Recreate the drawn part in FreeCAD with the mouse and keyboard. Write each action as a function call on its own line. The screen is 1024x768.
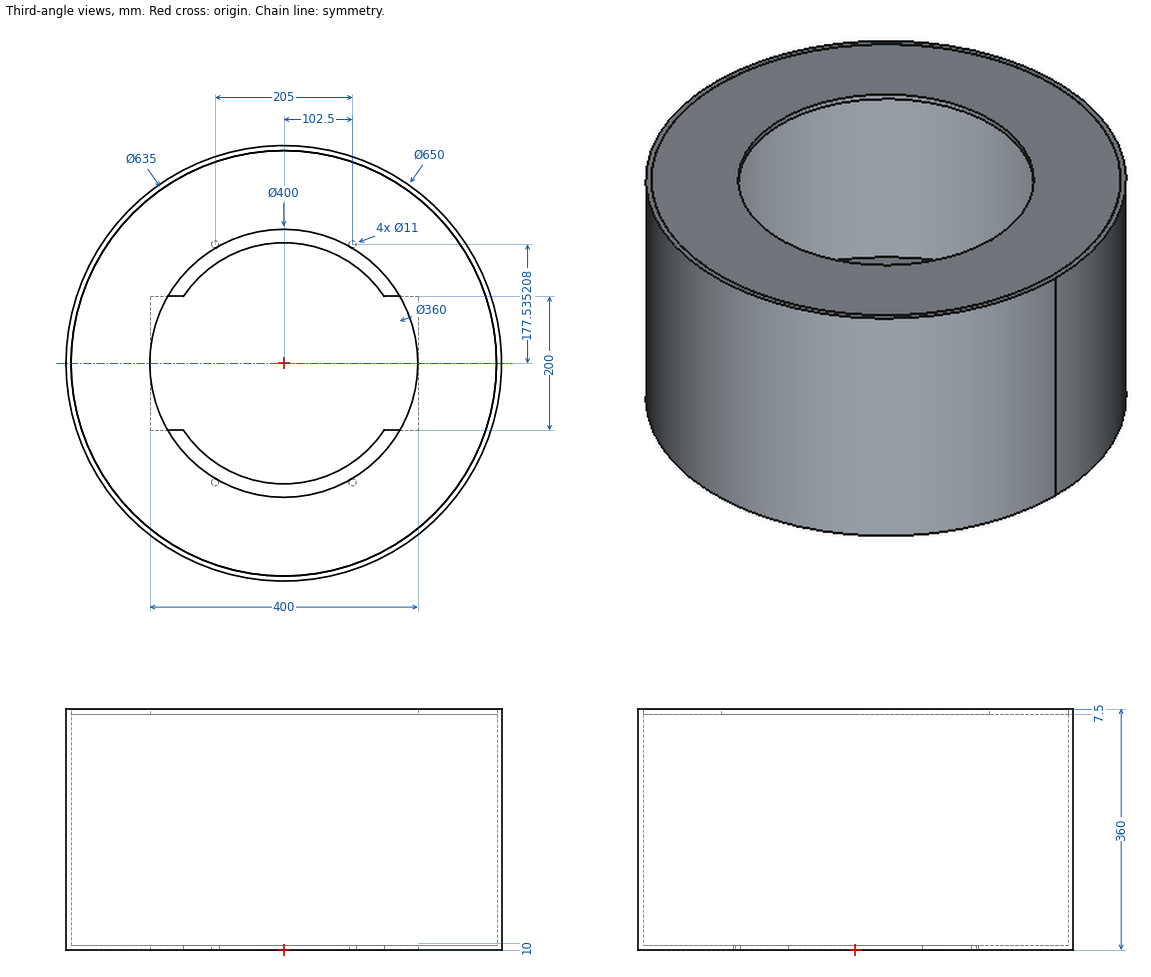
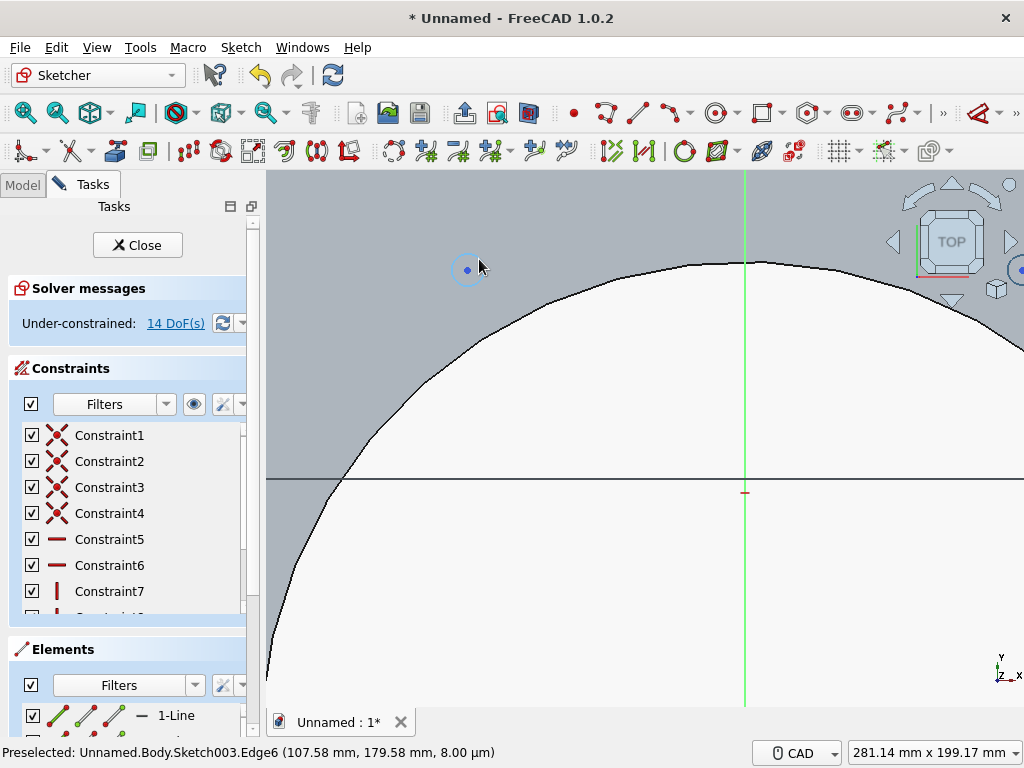
click(479, 259)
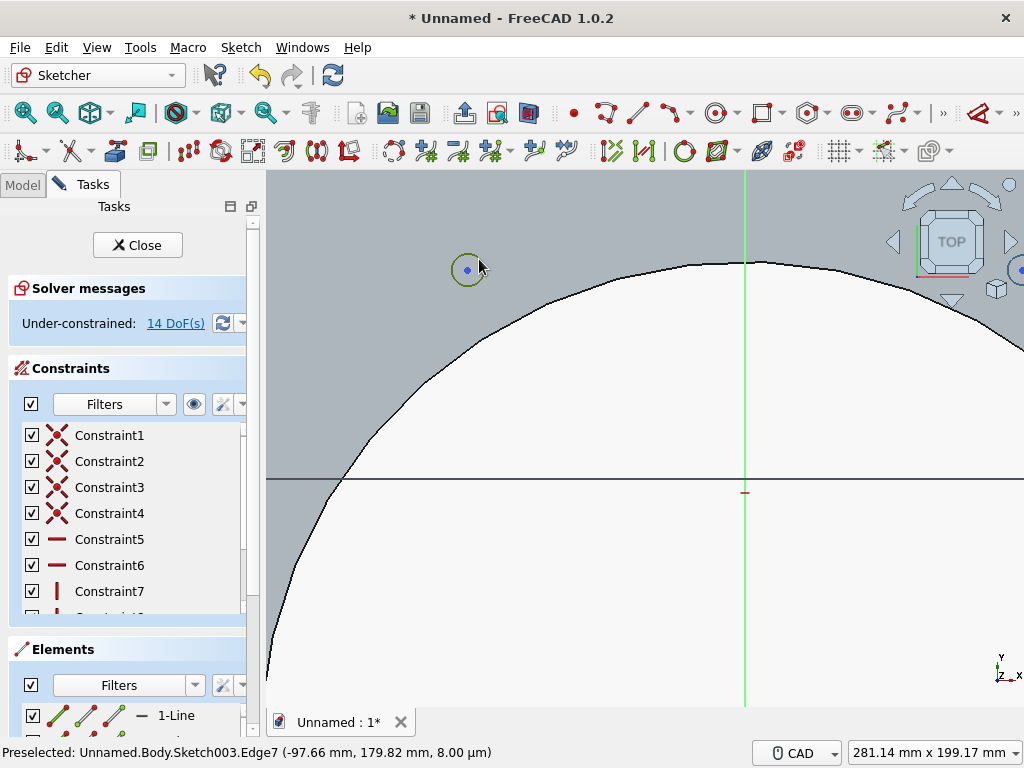
scroll(478, 259, down, 5)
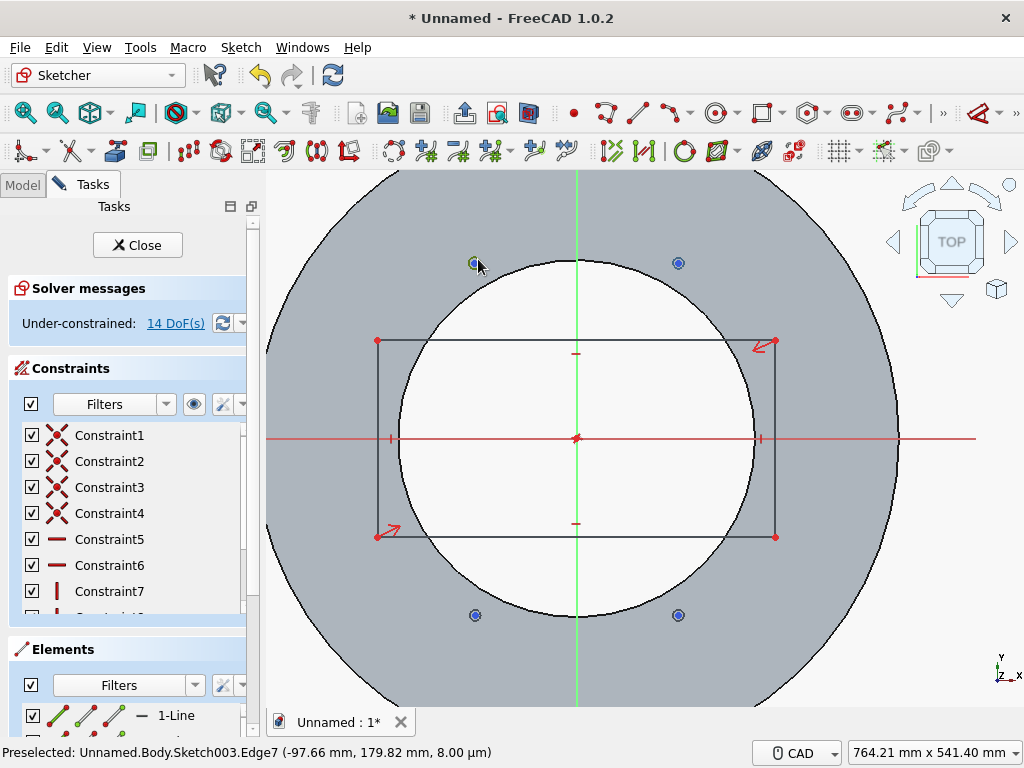
scroll(479, 612, up, 5)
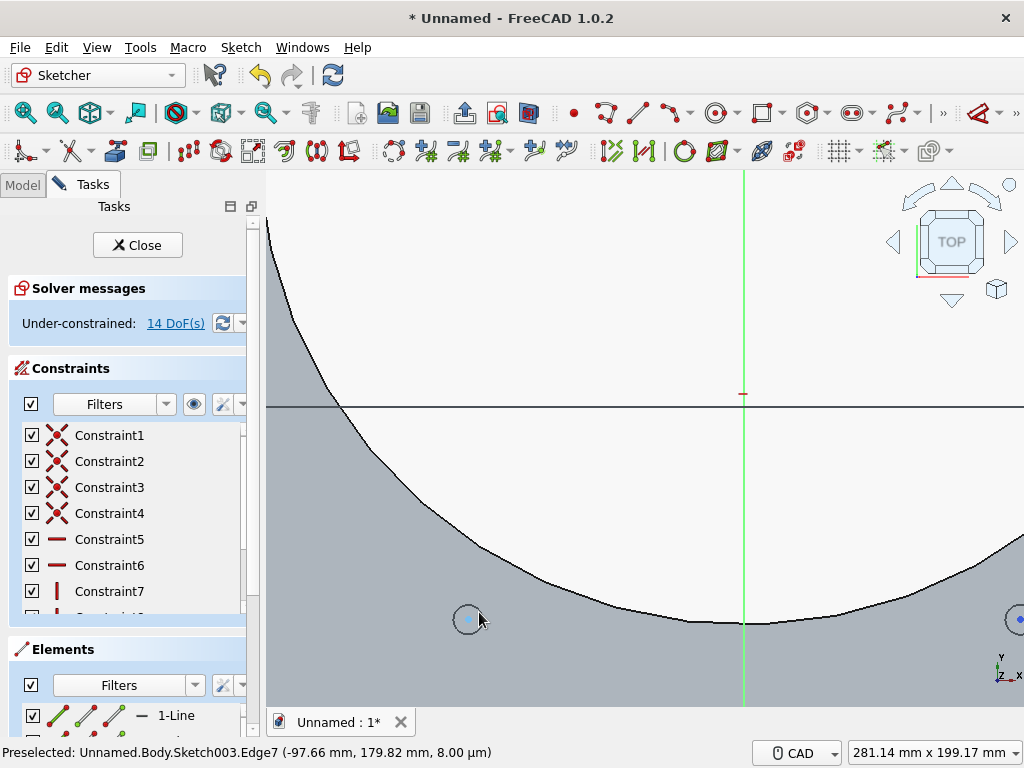
click(478, 609)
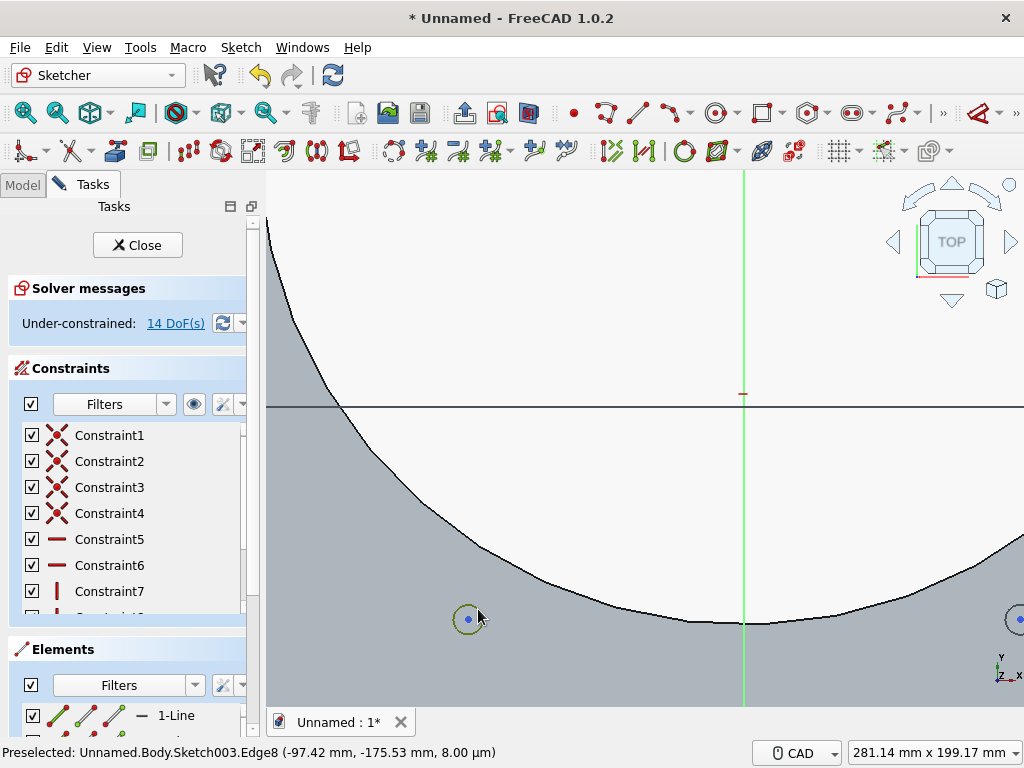
scroll(479, 613, down, 5)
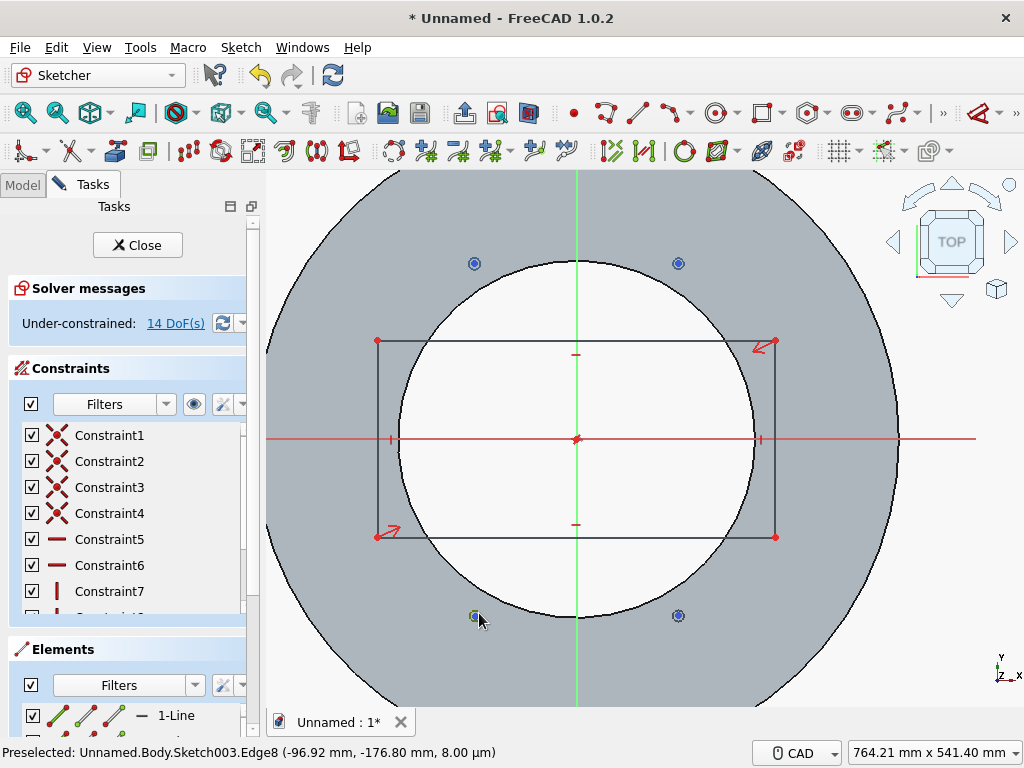
scroll(682, 612, up, 5)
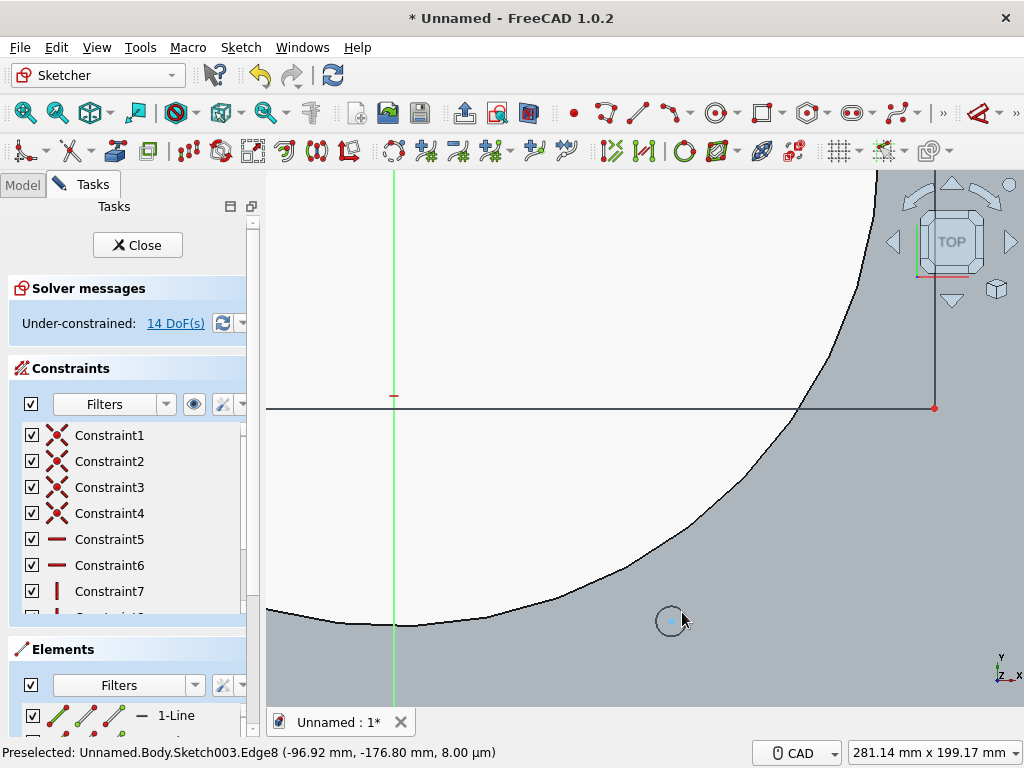
click(682, 611)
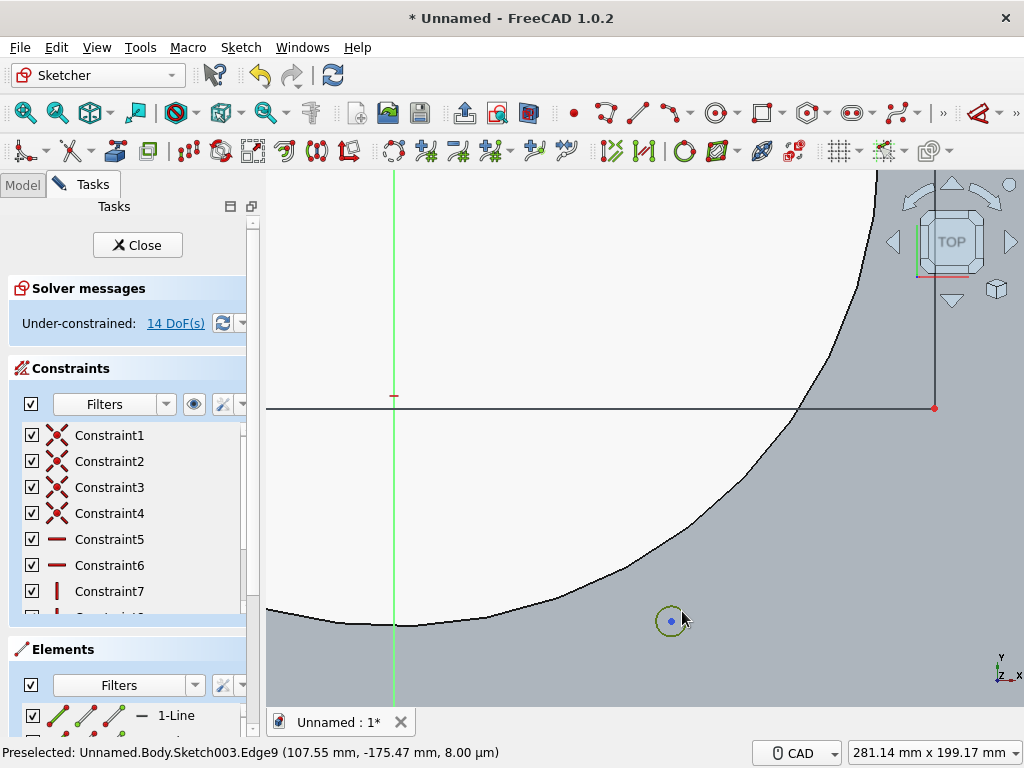
key(e)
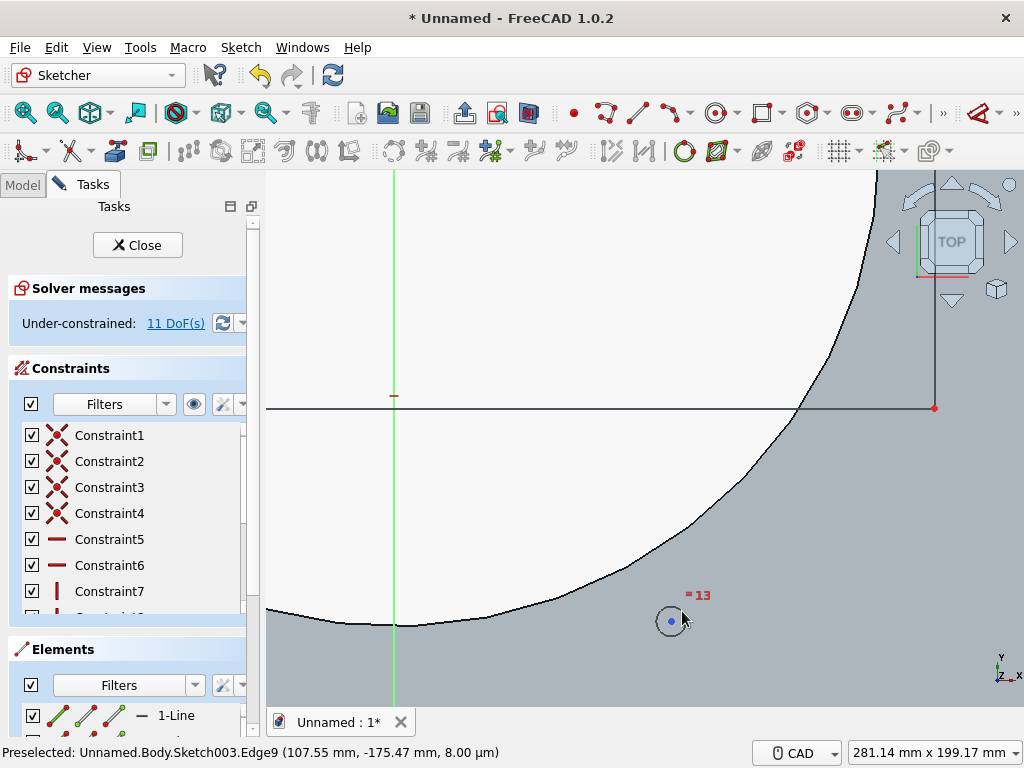
scroll(683, 612, down, 5)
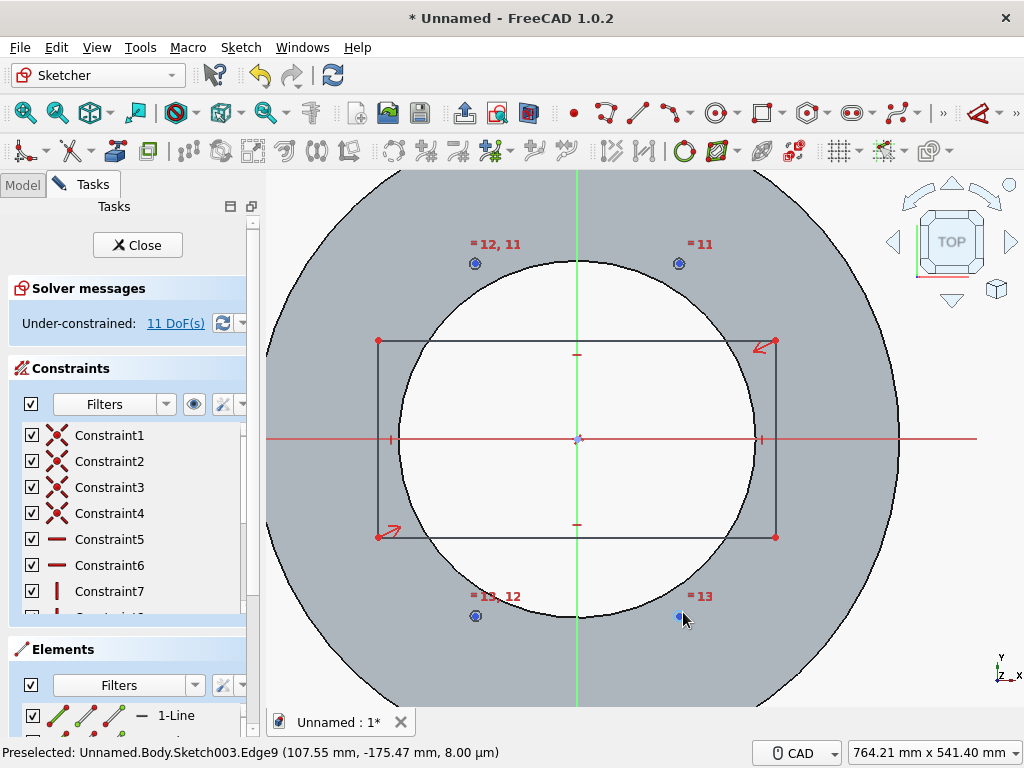
click(679, 264)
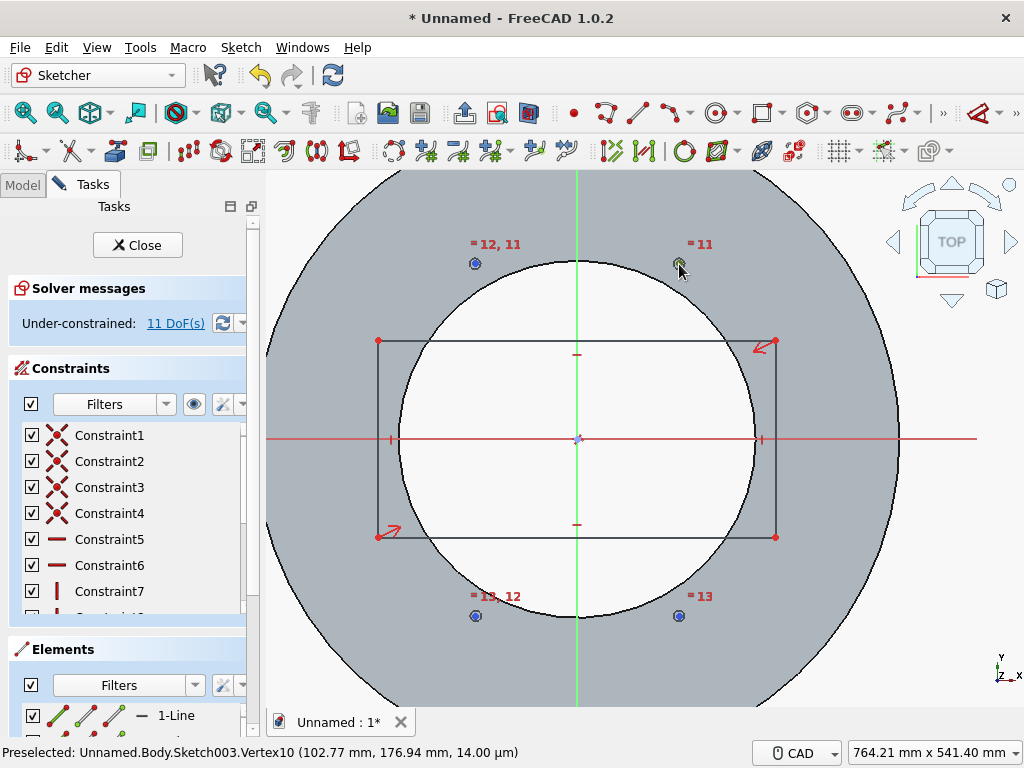
click(475, 264)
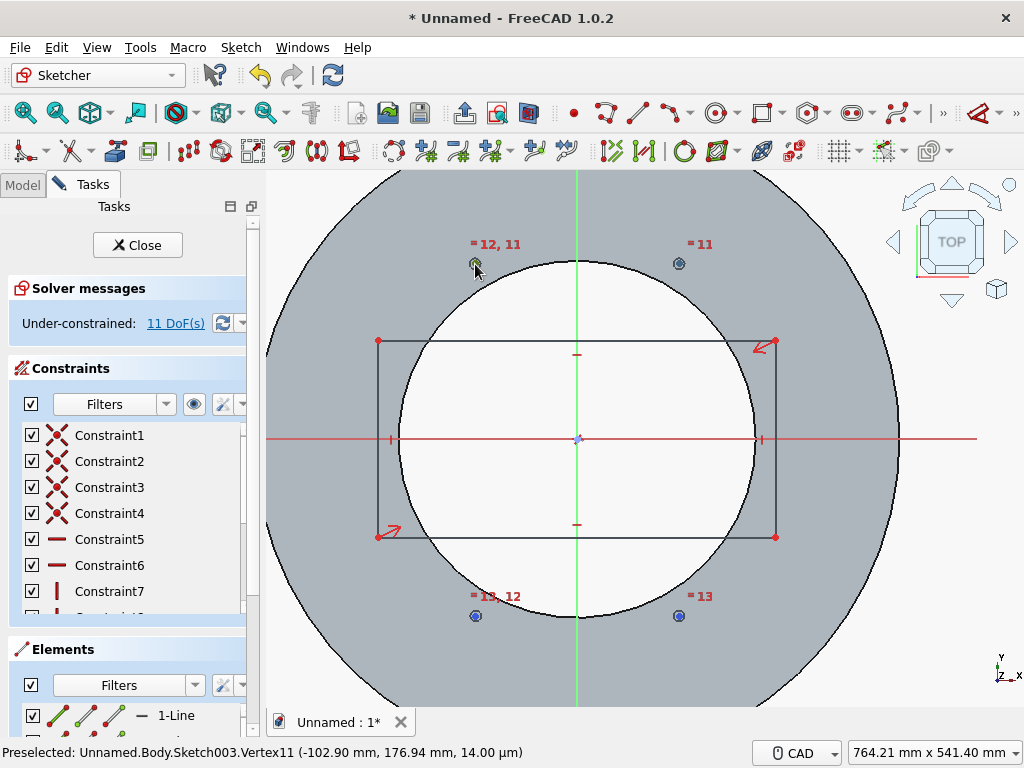
key(h)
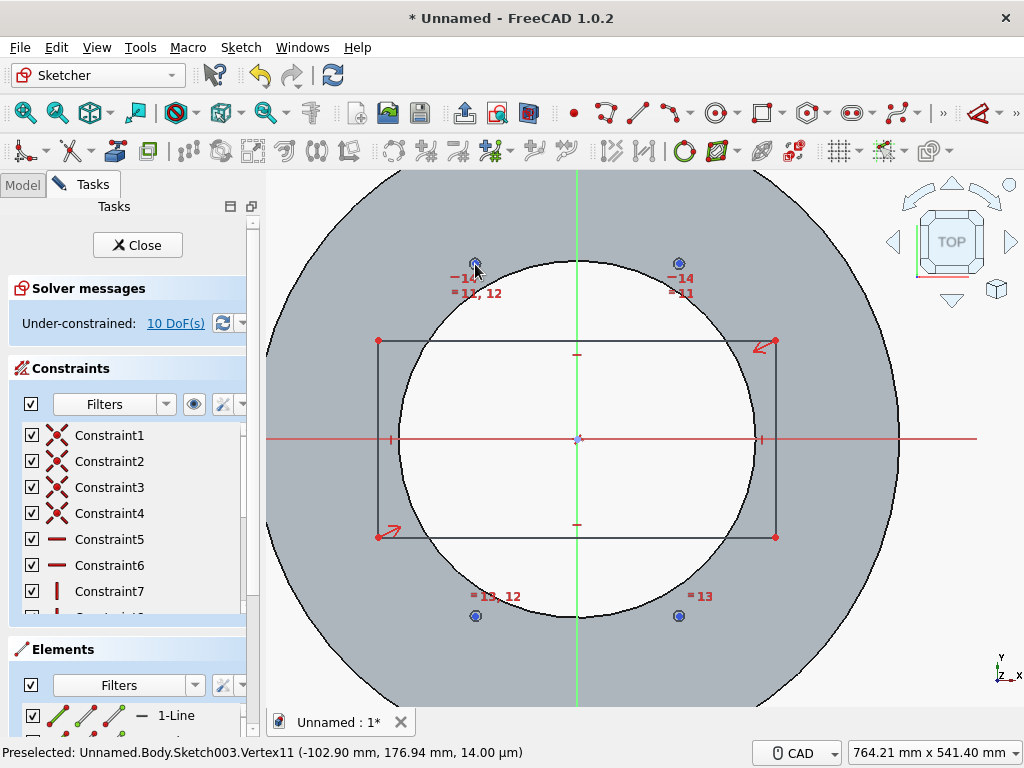
click(476, 616)